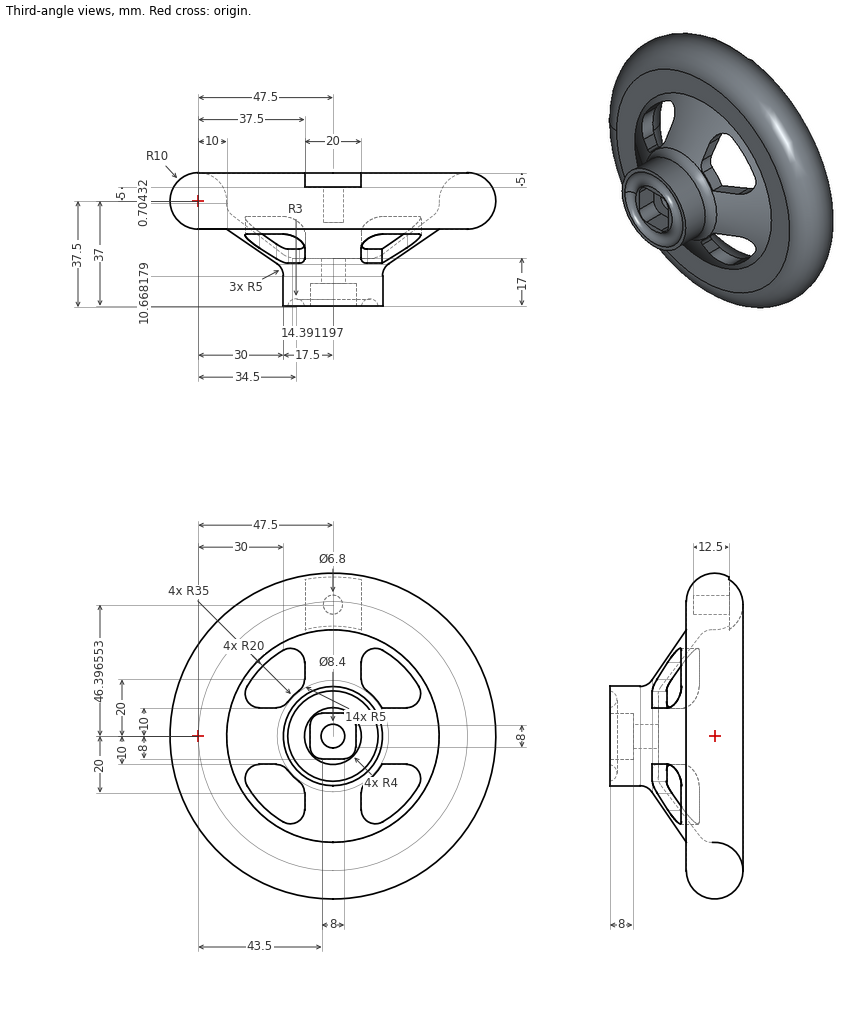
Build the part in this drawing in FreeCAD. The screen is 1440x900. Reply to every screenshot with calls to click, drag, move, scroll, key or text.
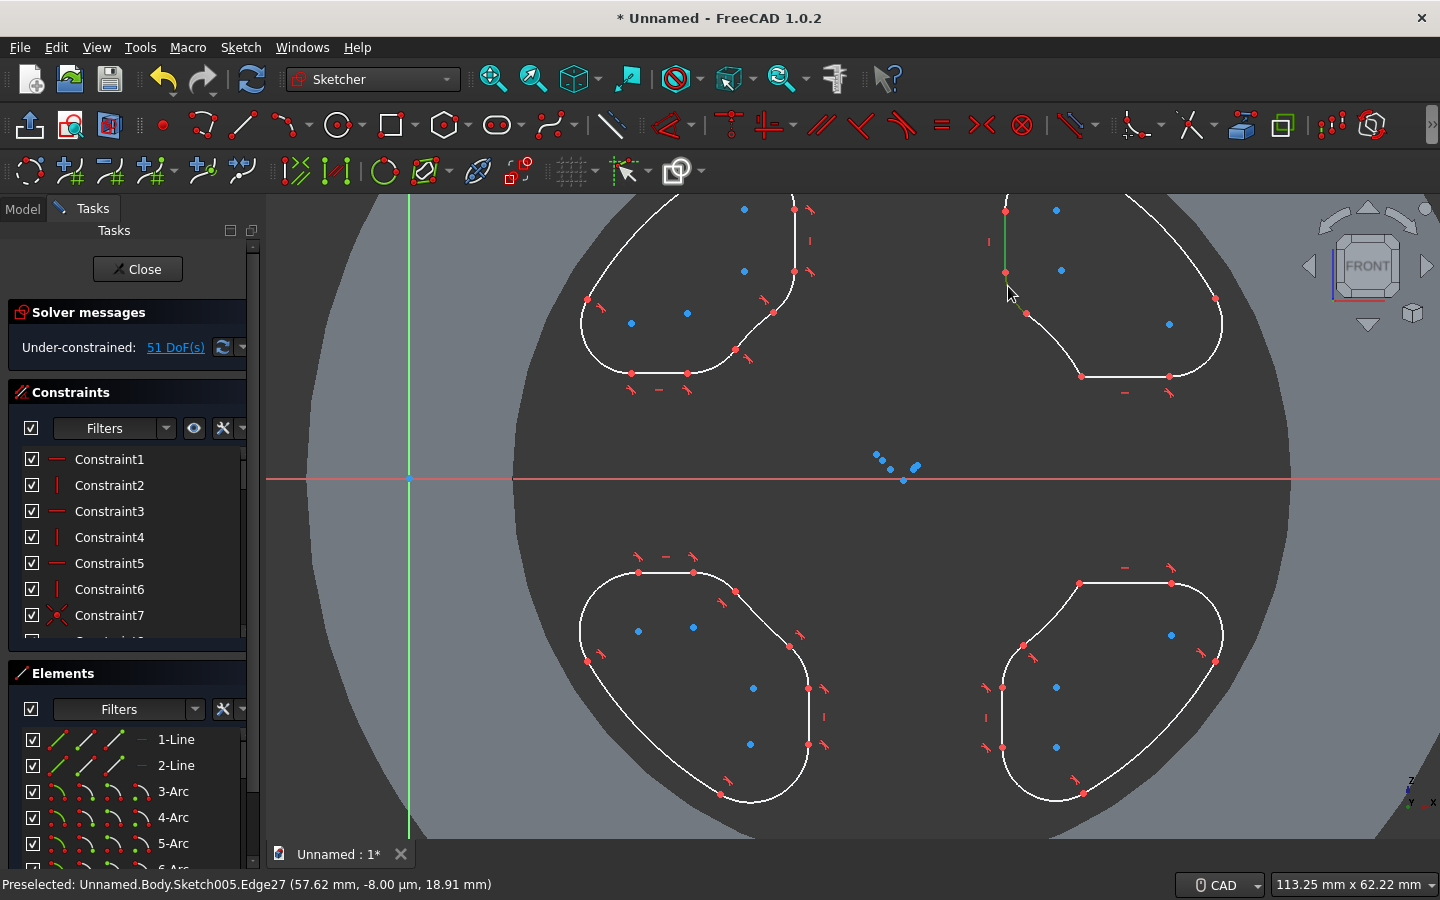
click(902, 126)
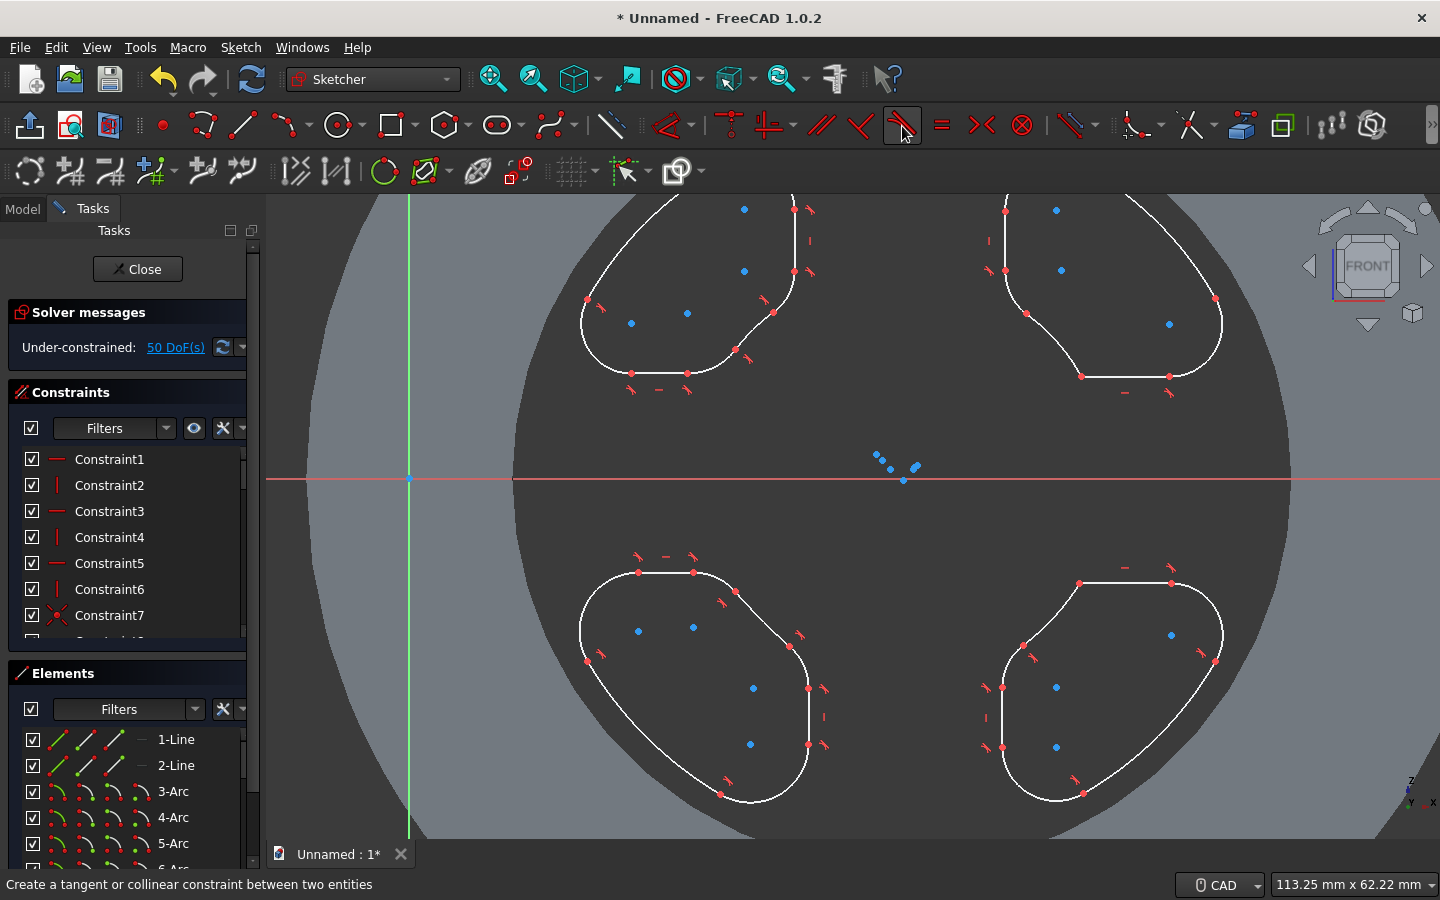
click(1005, 252)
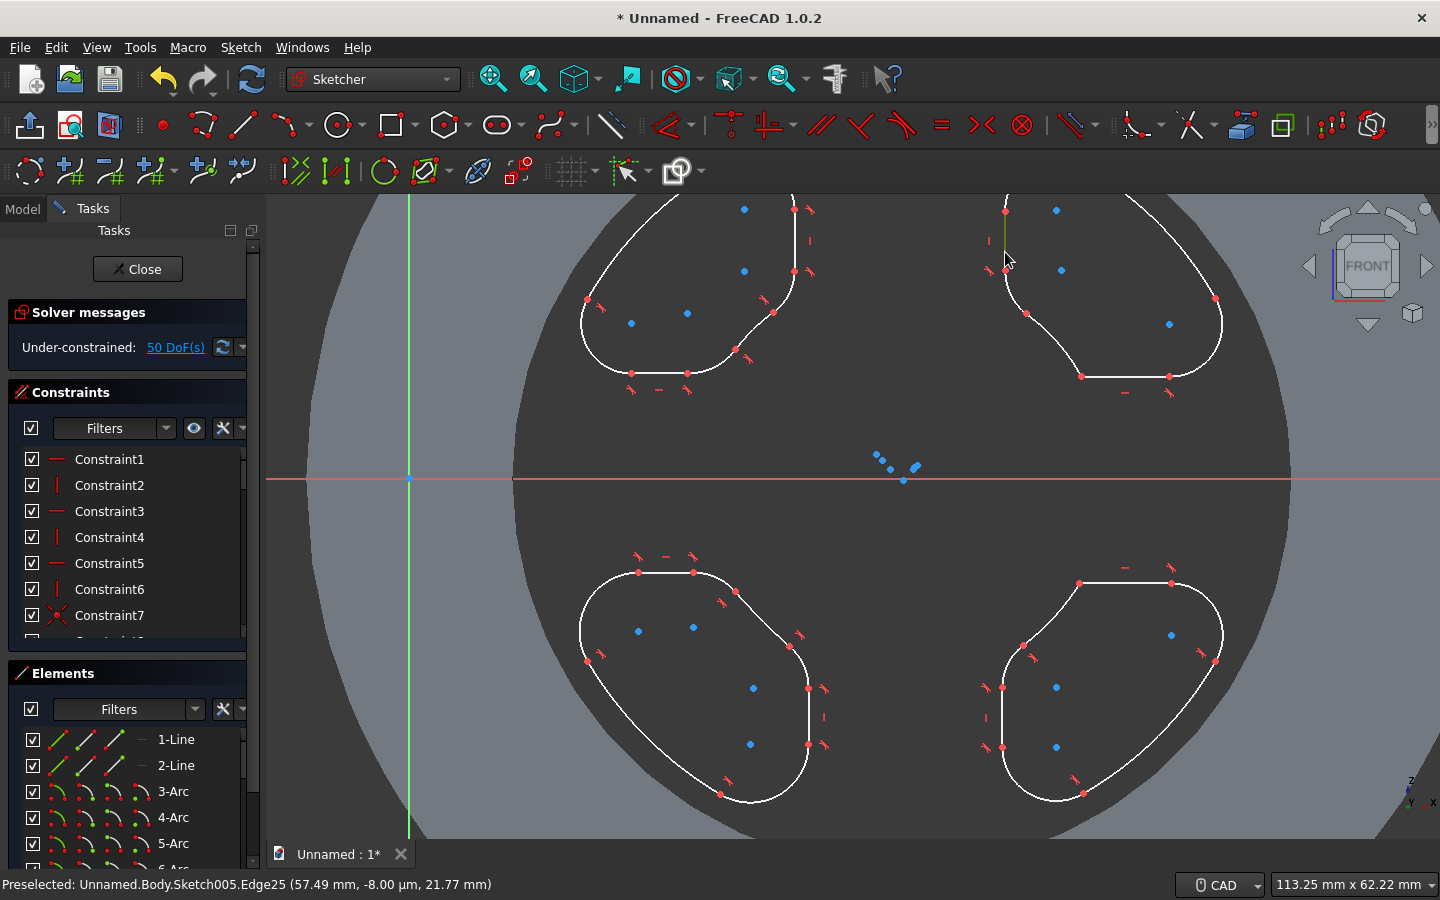
scroll(727, 593, down, 2)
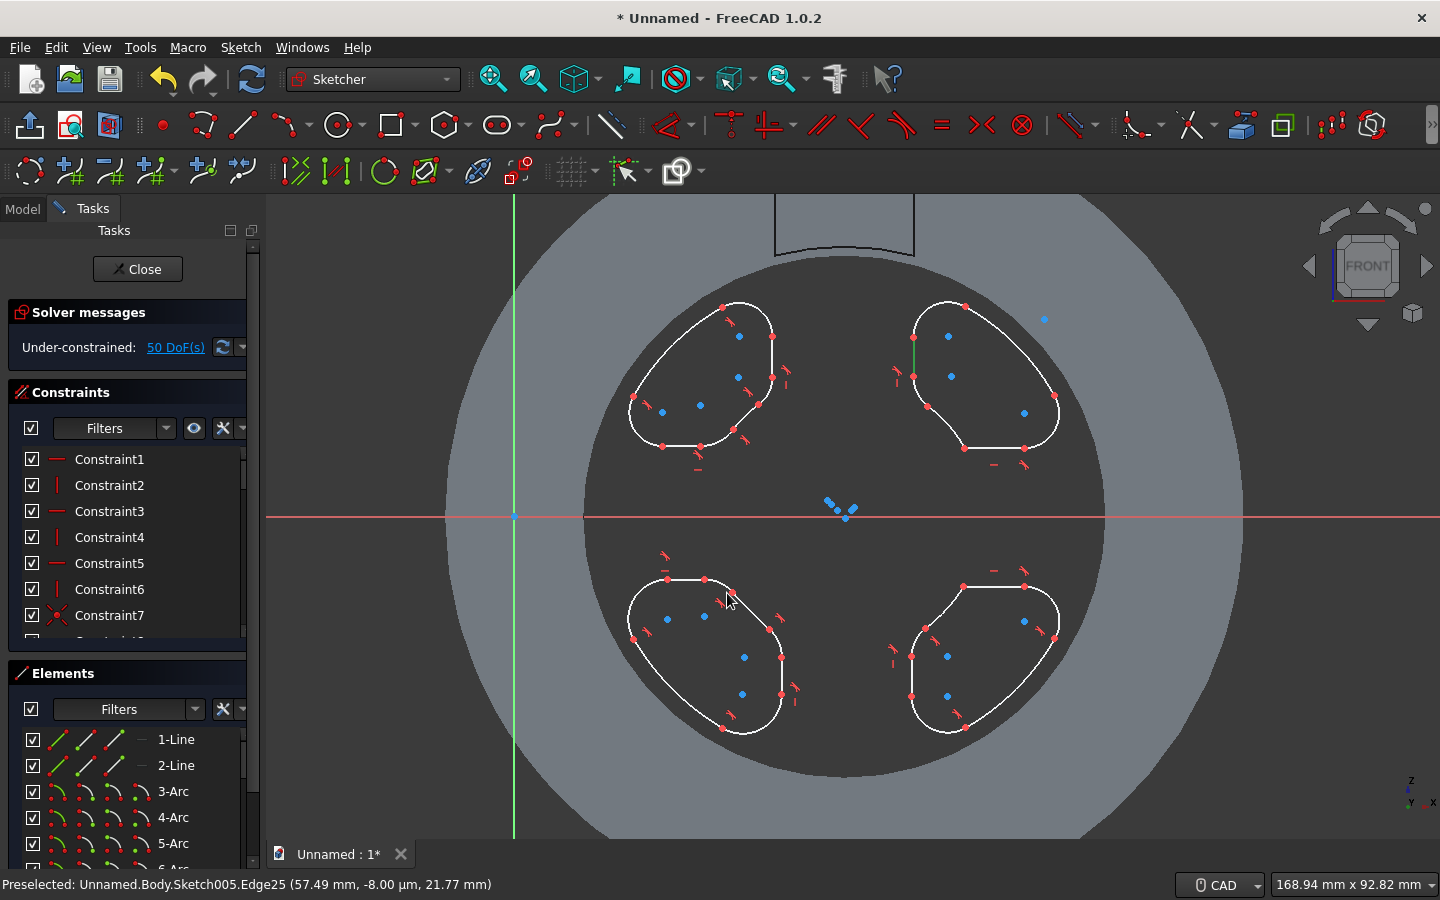
click(945, 302)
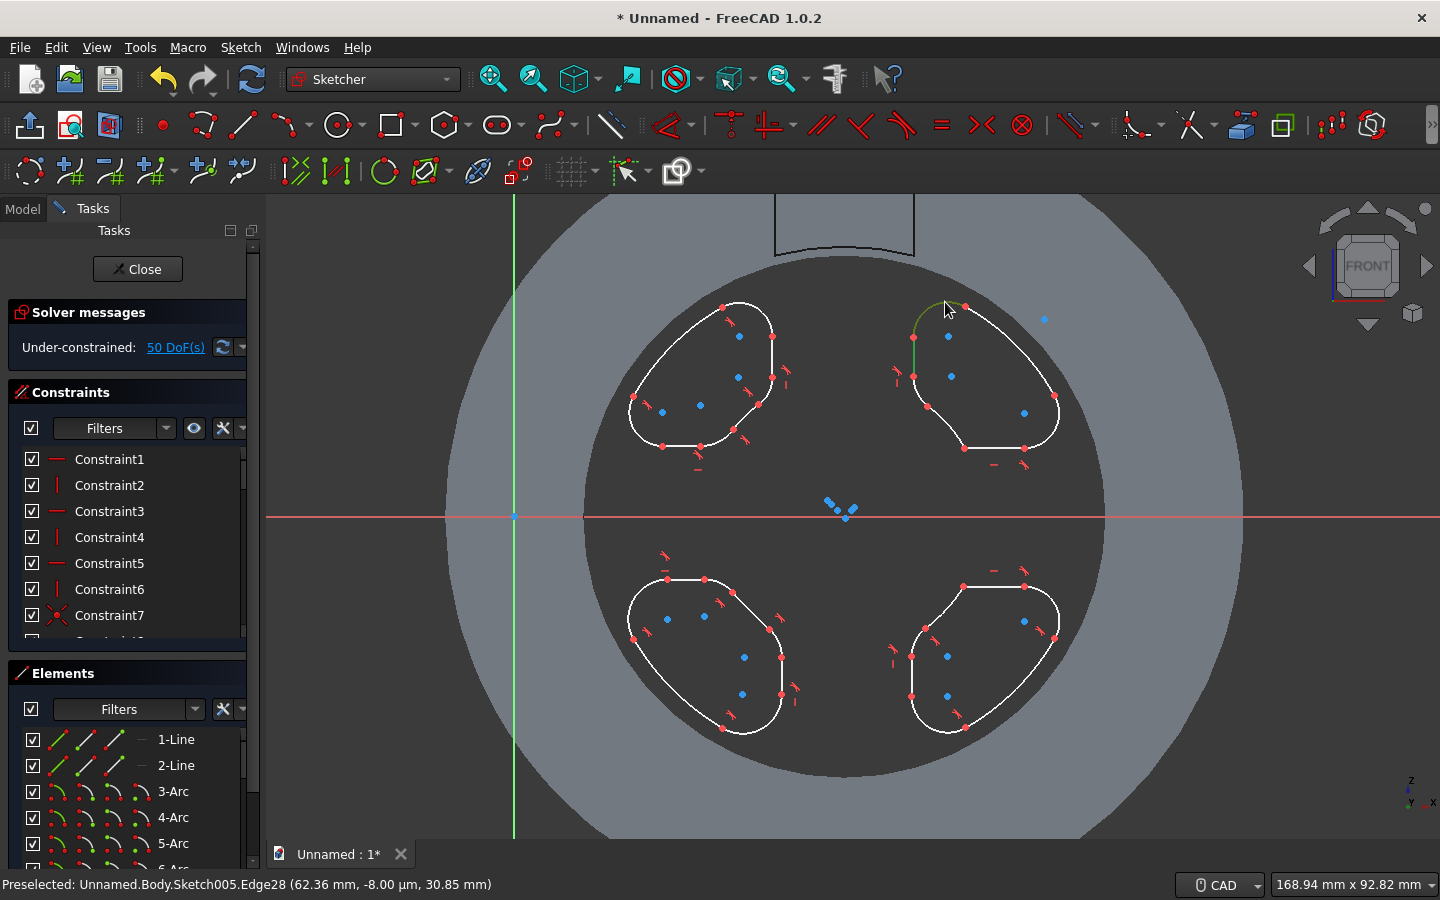
click(902, 126)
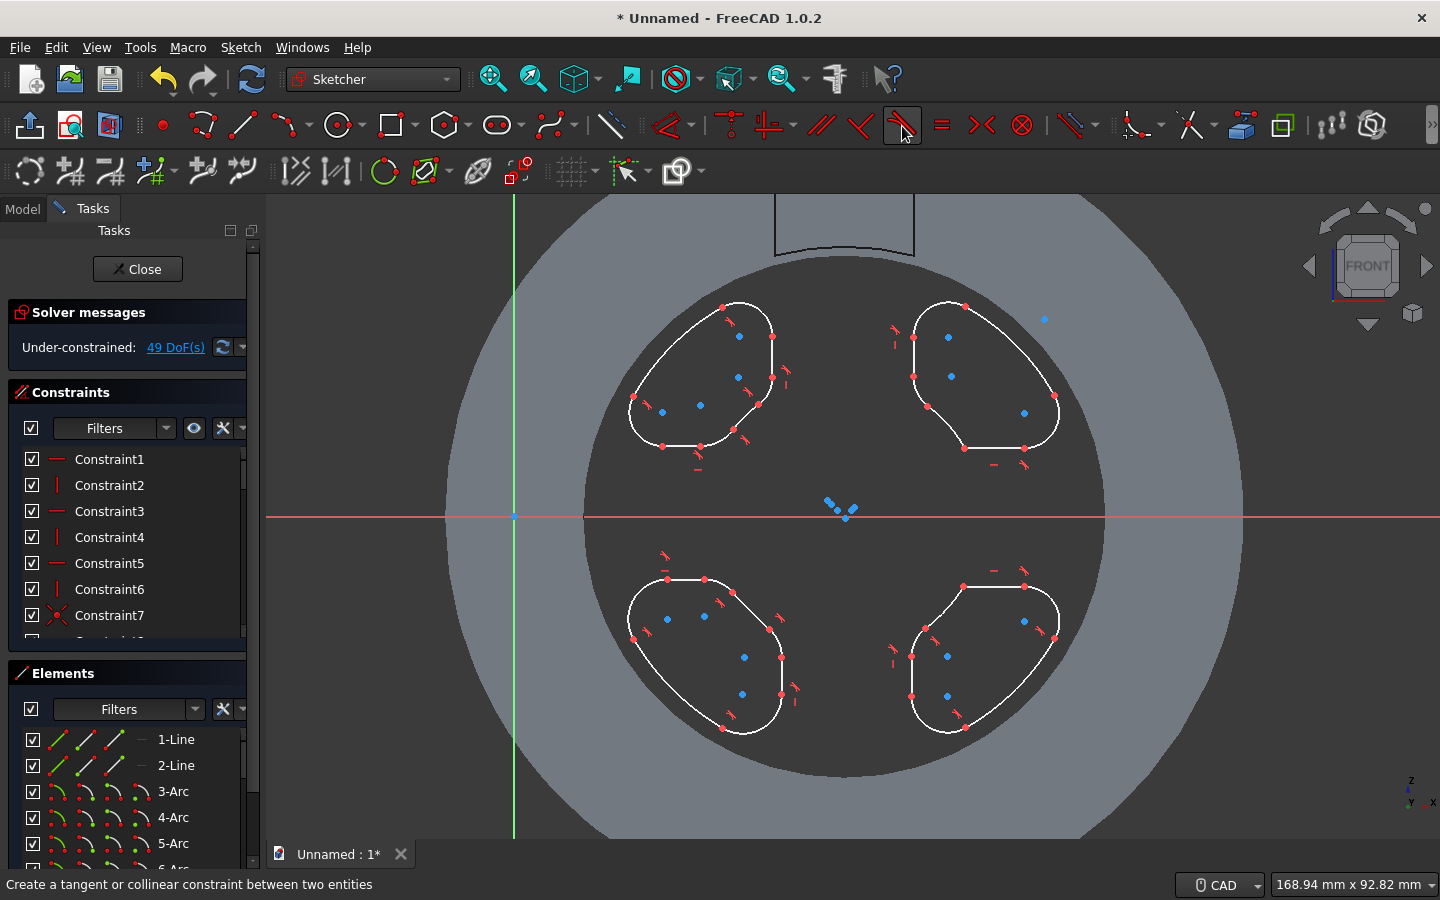
click(956, 434)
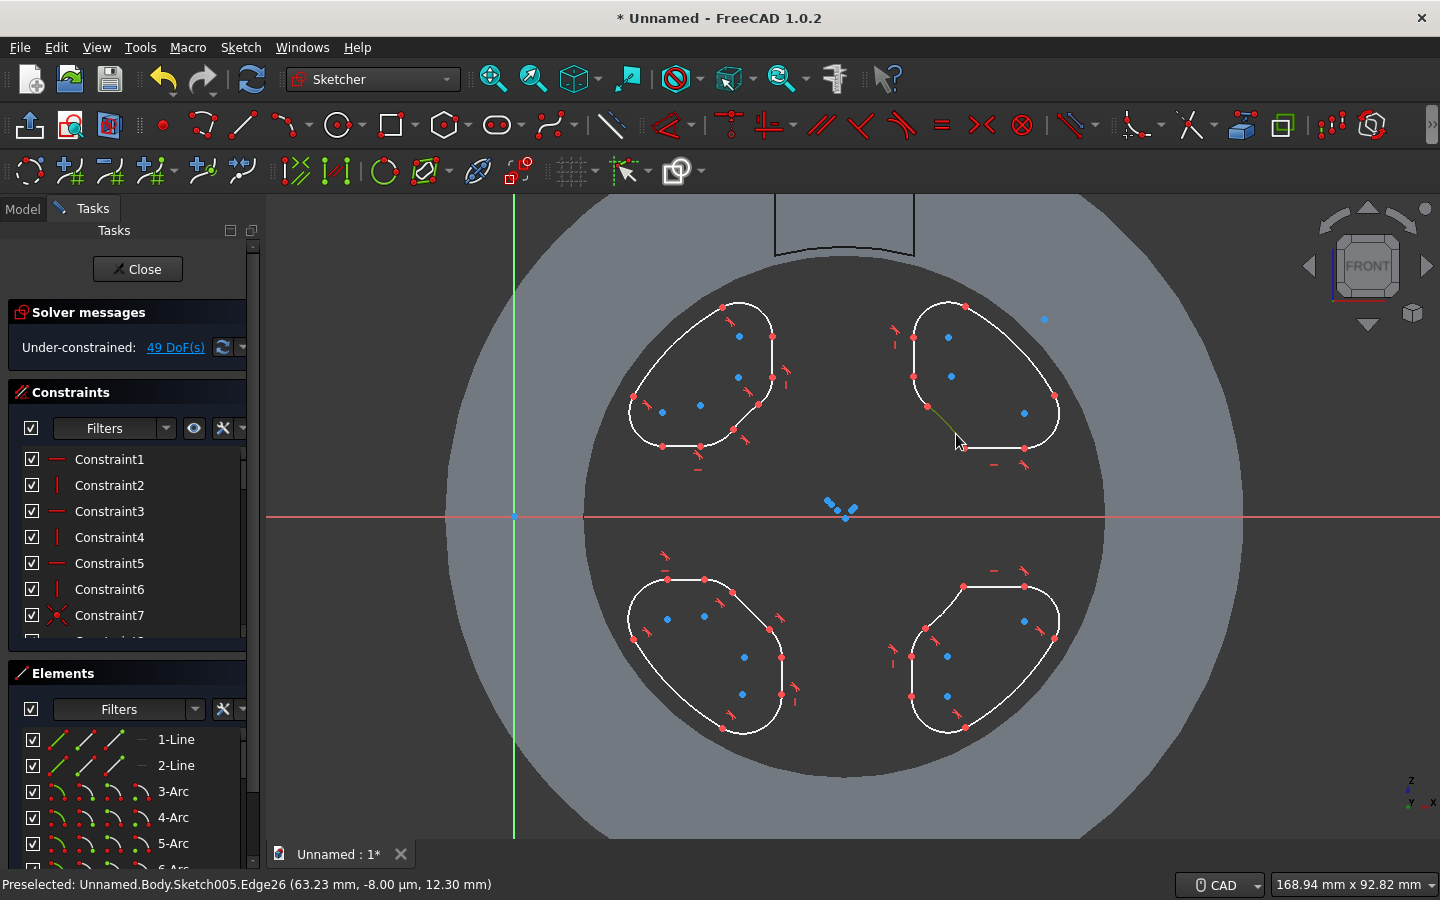
scroll(915, 387, up, 2)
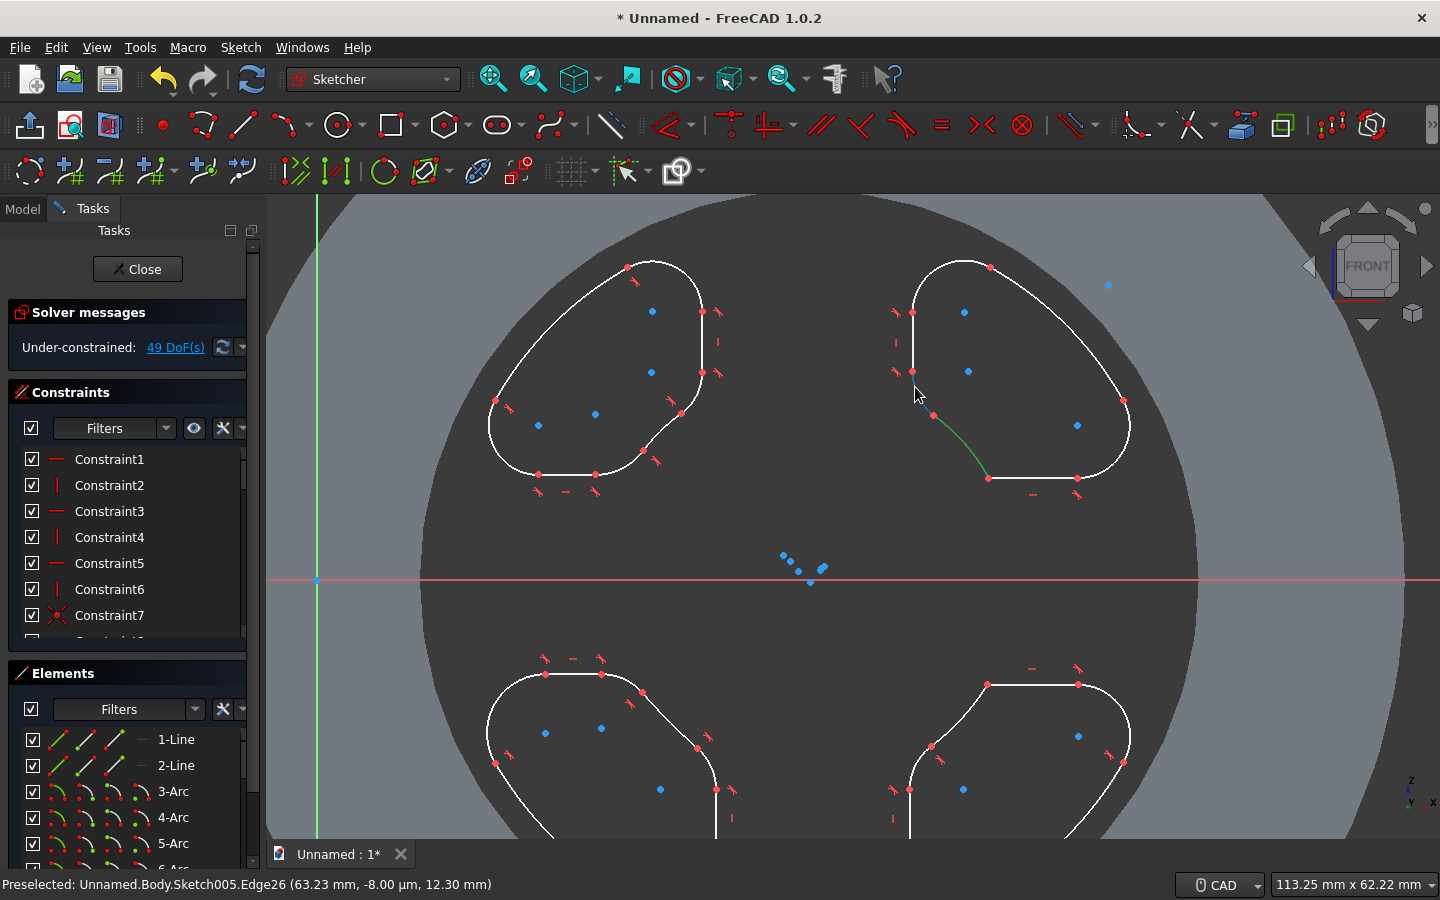
click(915, 387)